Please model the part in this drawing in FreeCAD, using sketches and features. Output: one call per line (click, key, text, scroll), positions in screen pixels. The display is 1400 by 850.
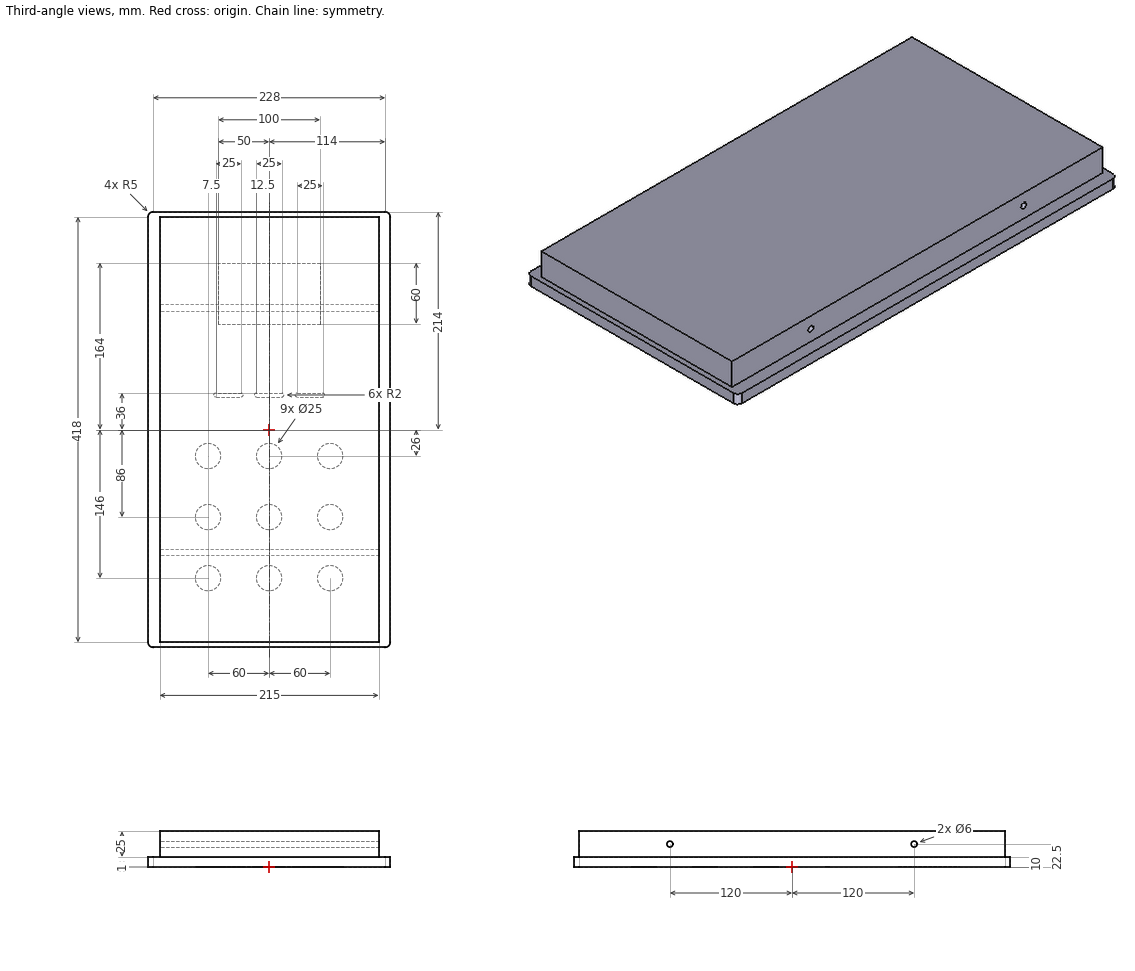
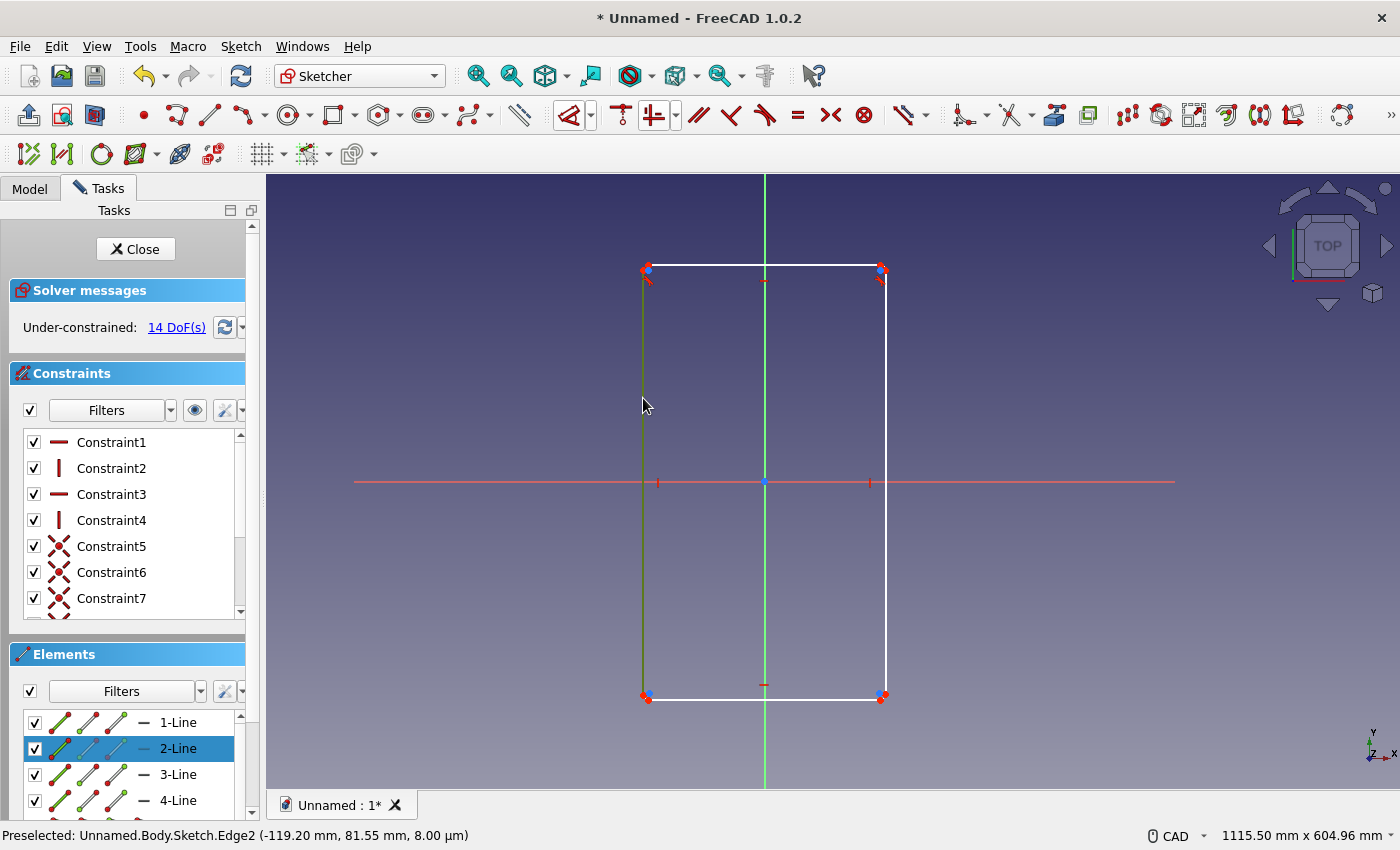
scroll(645, 267, up, 7)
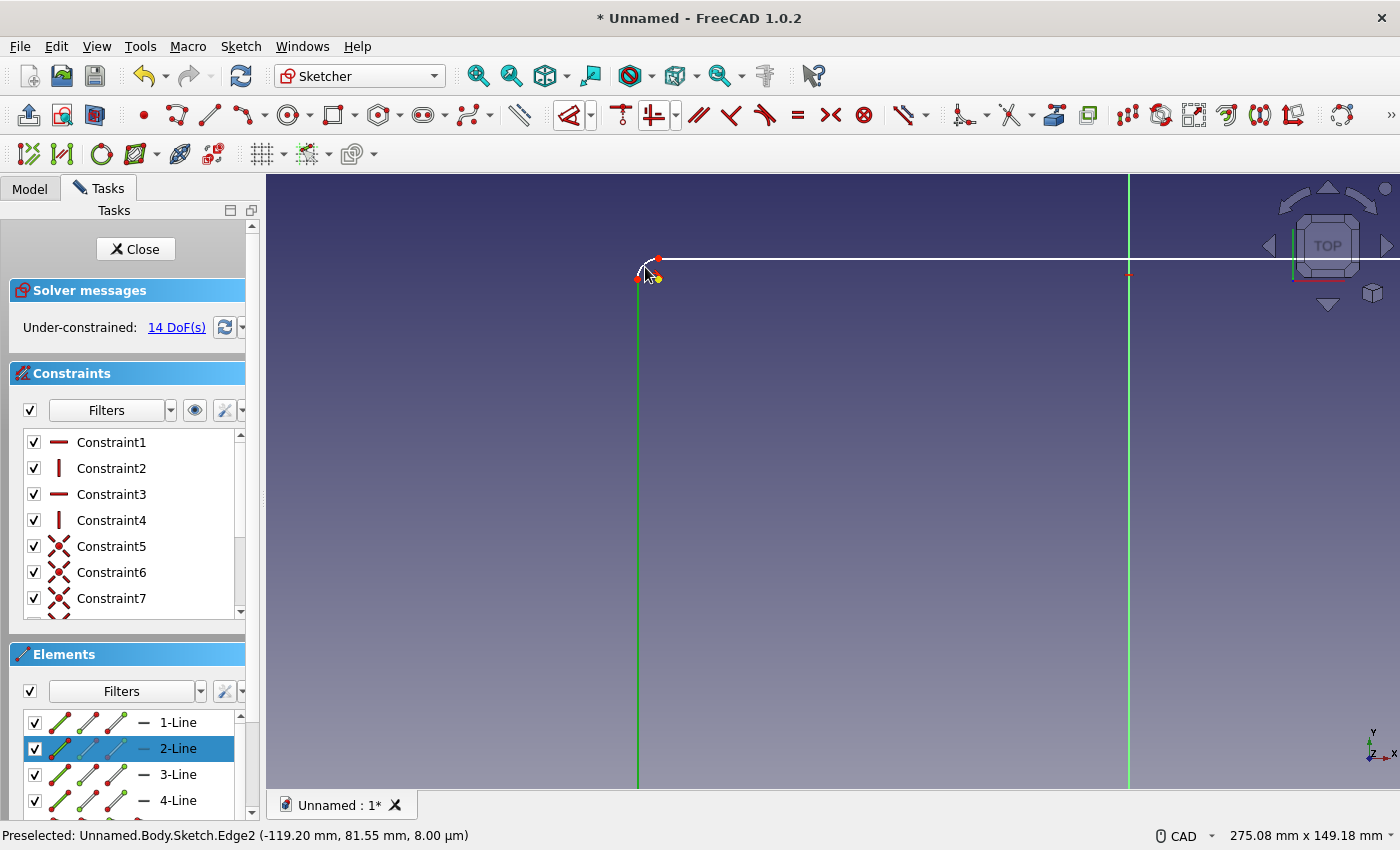
click(644, 265)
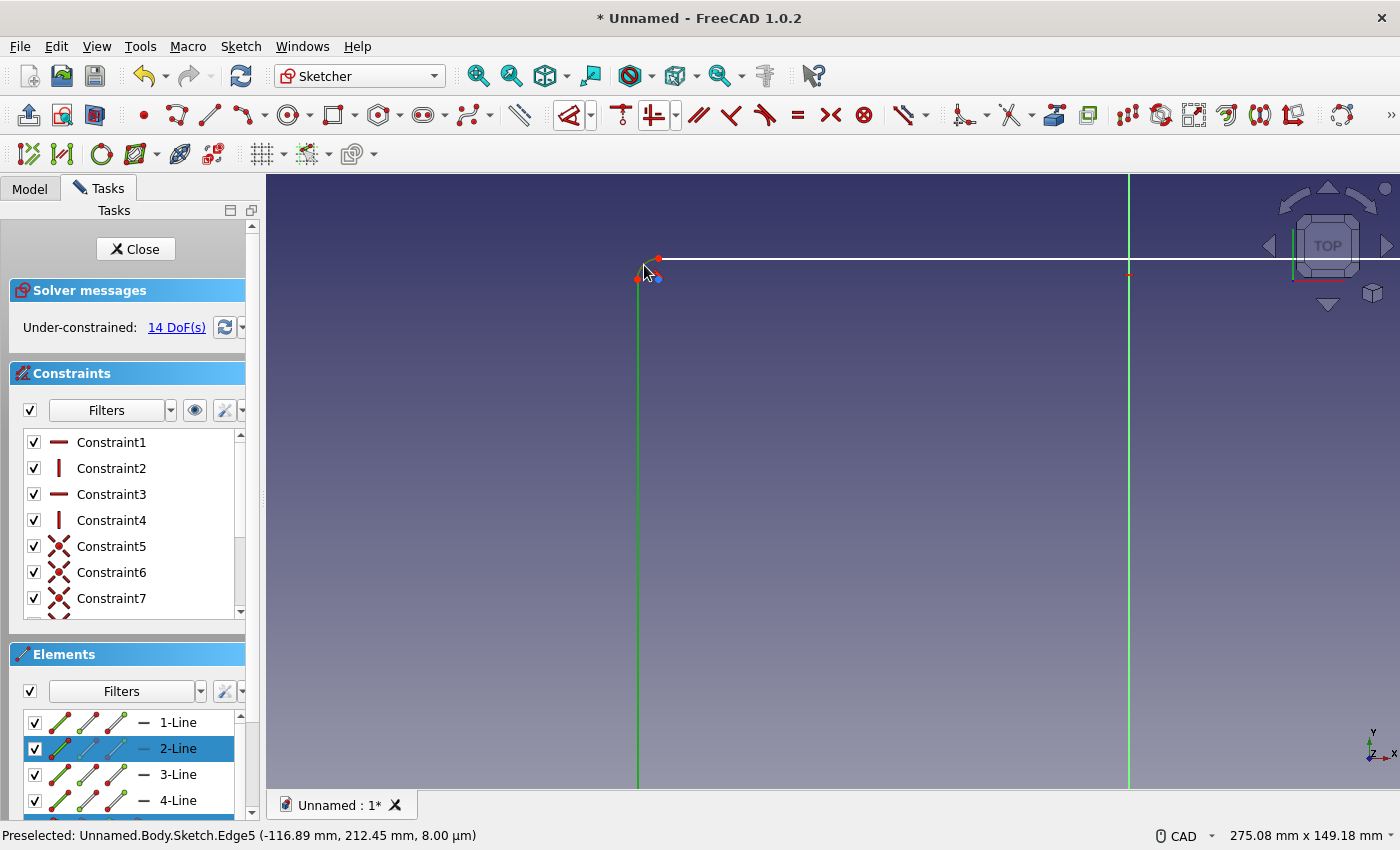
click(765, 116)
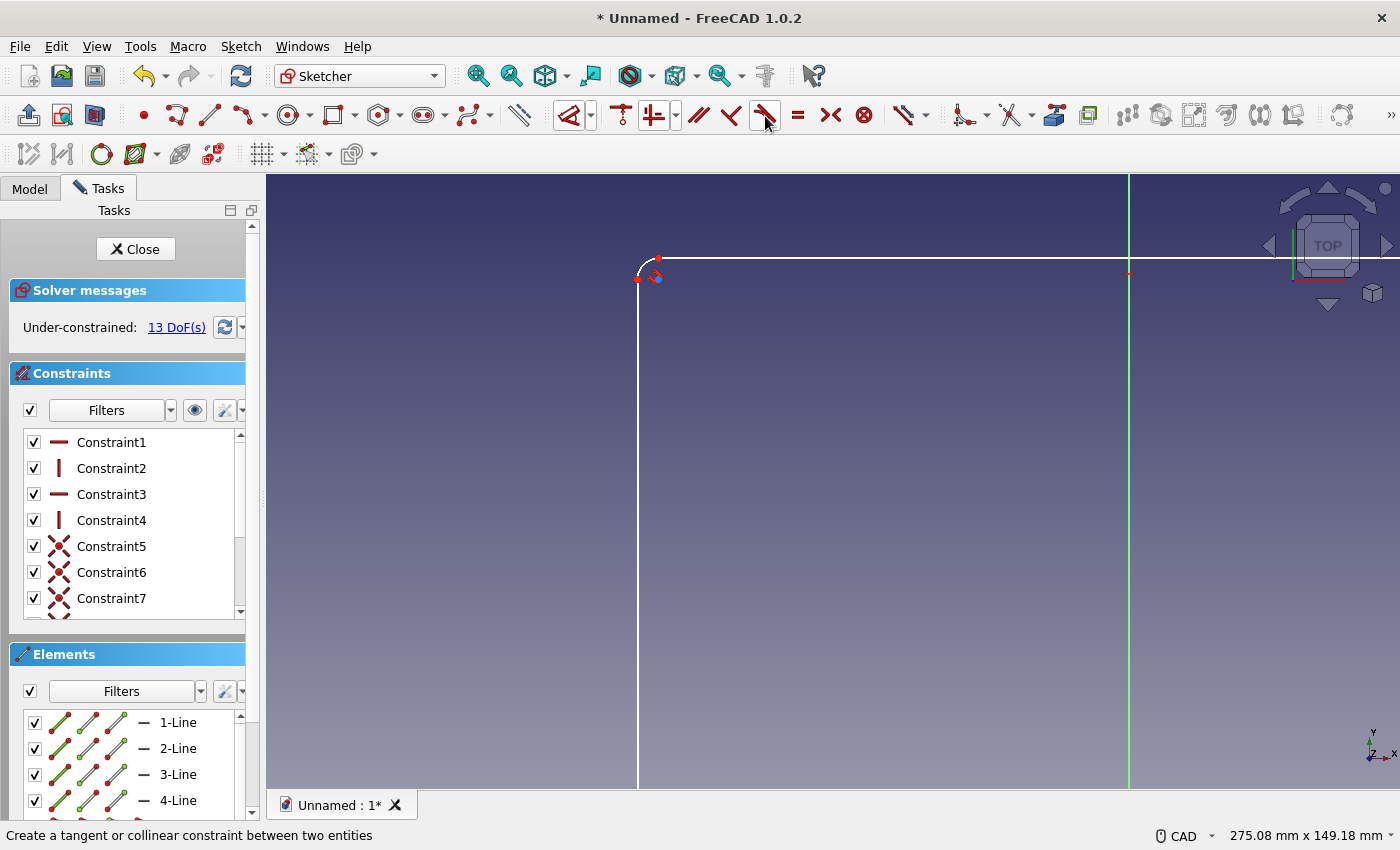
scroll(645, 267, down, 7)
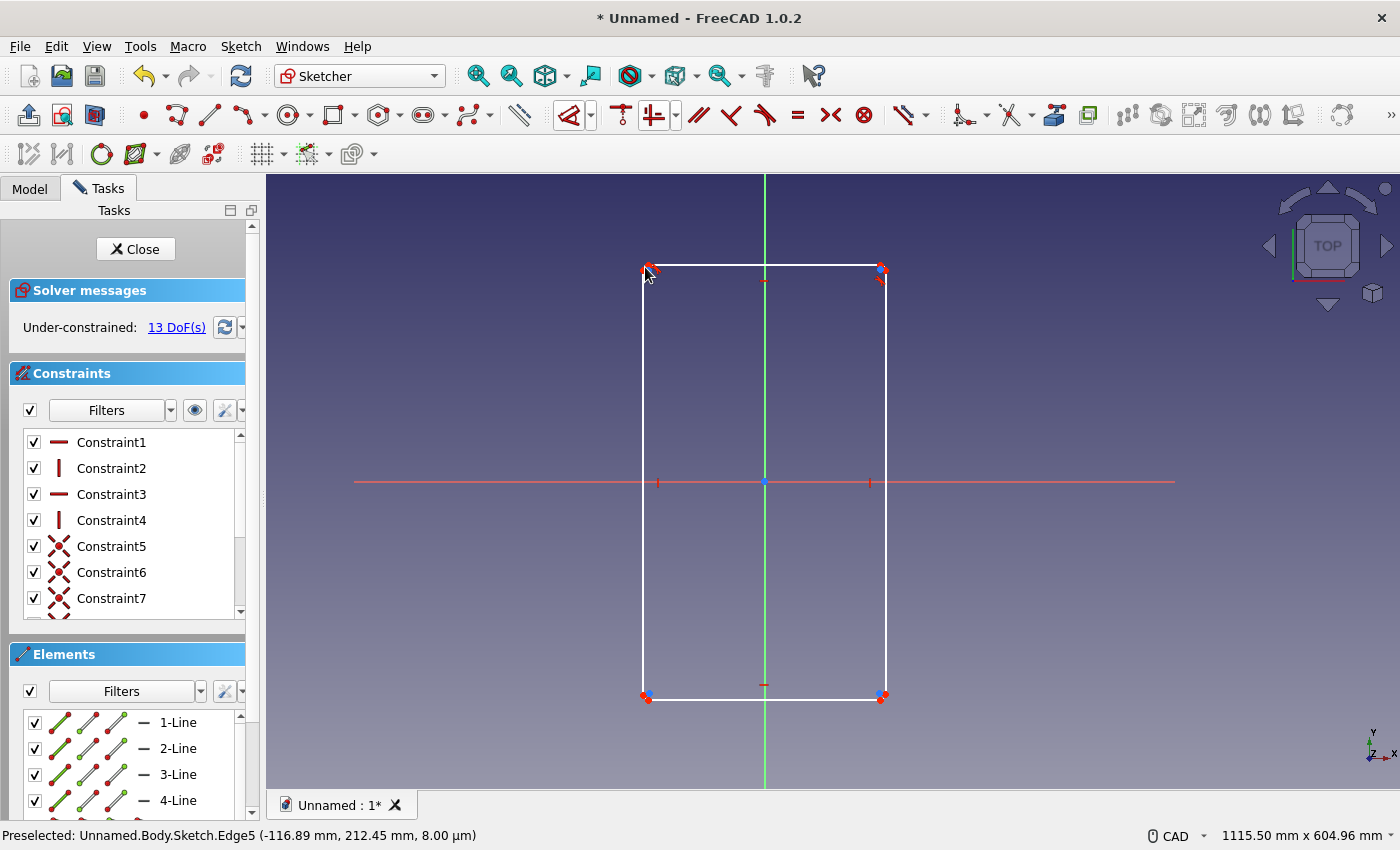
click(643, 355)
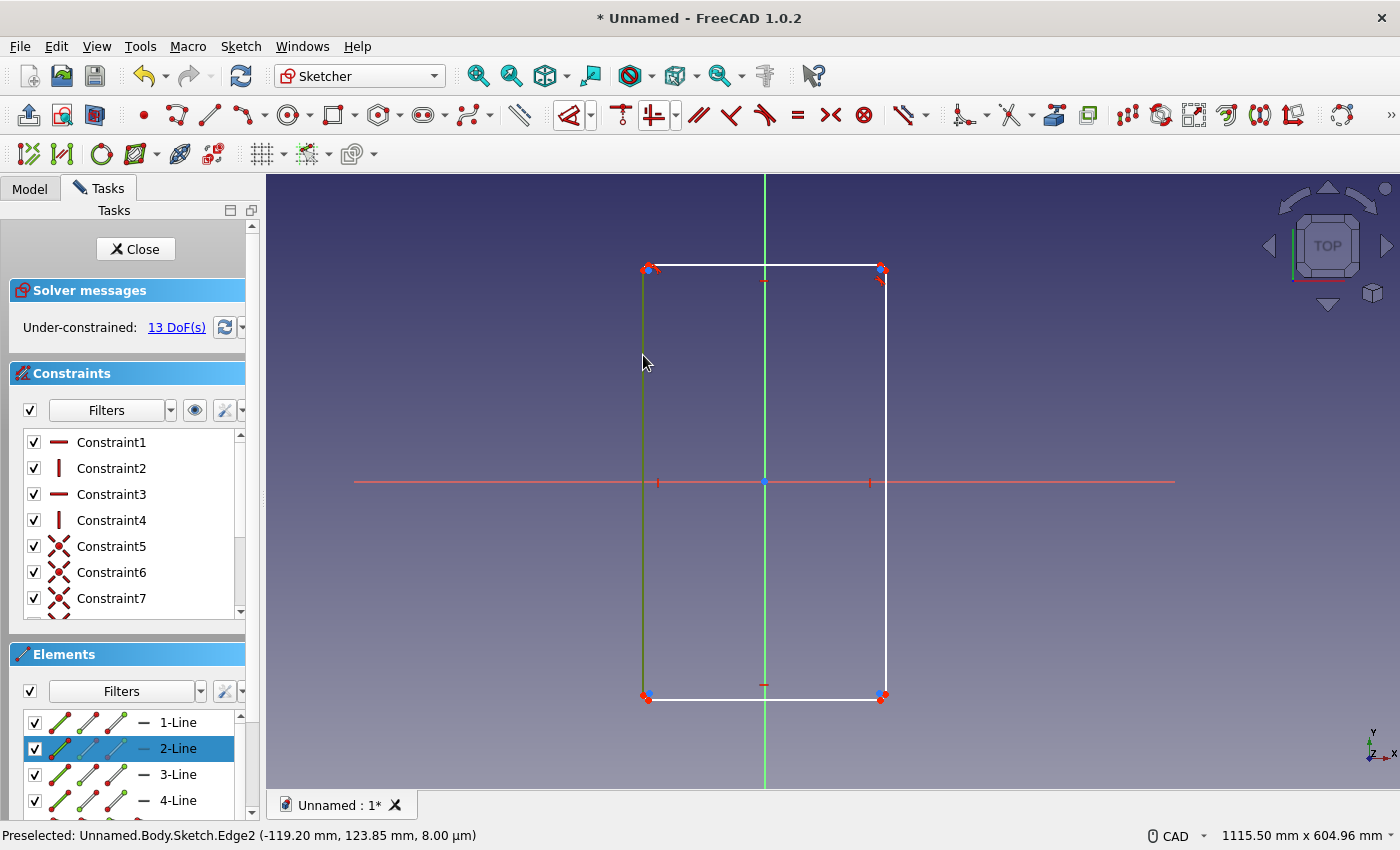
scroll(645, 698, up, 7)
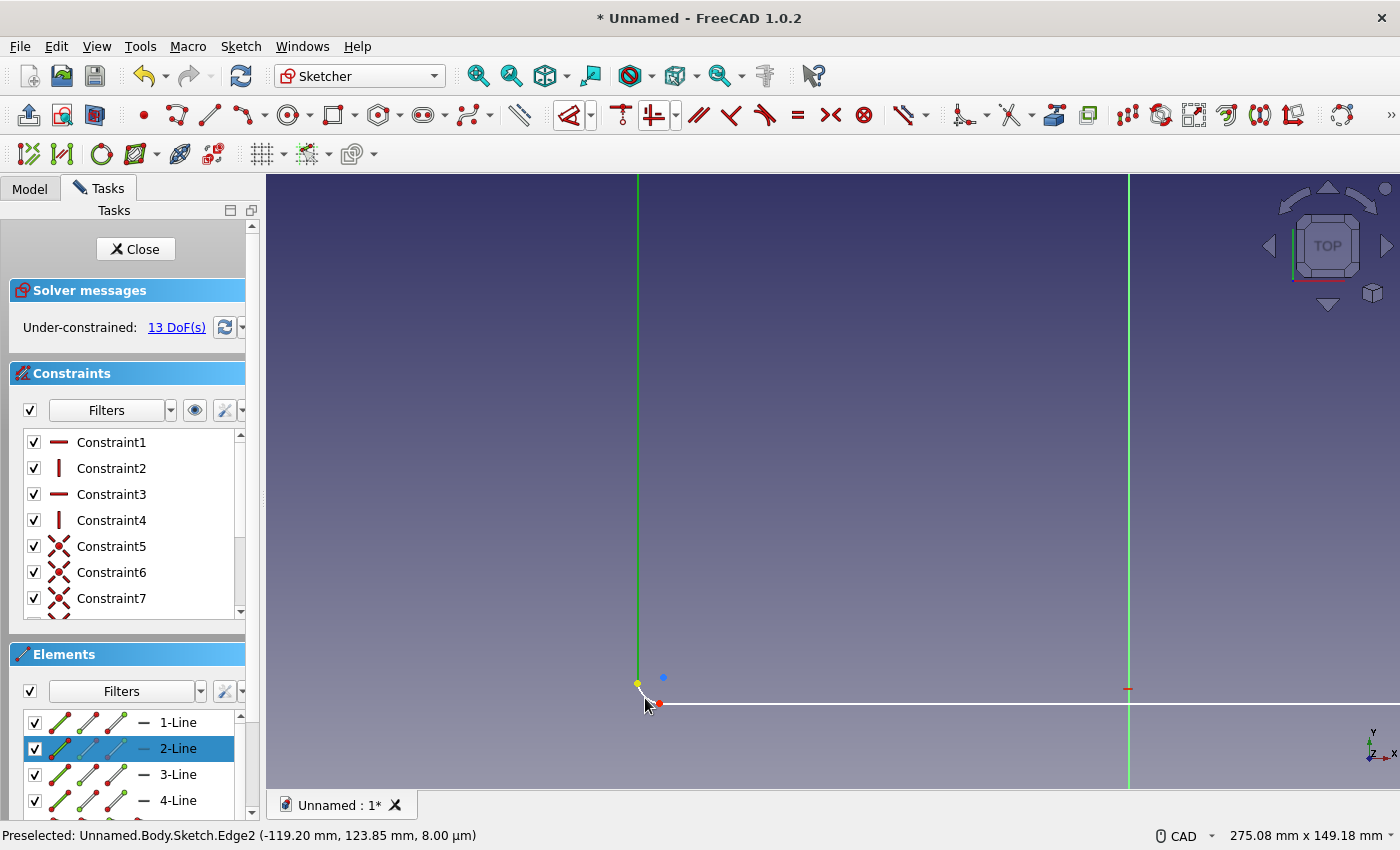
click(646, 697)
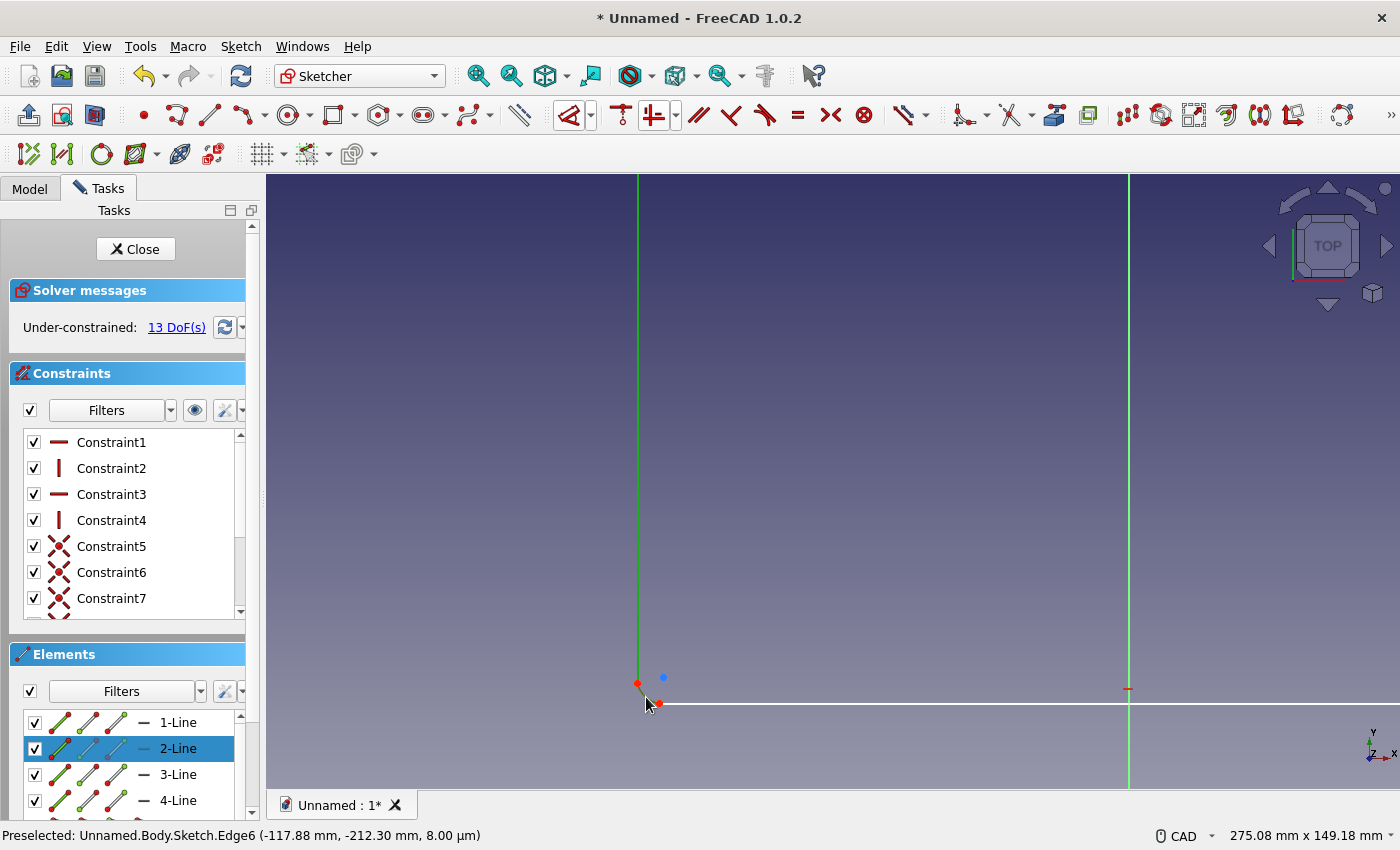
click(765, 116)